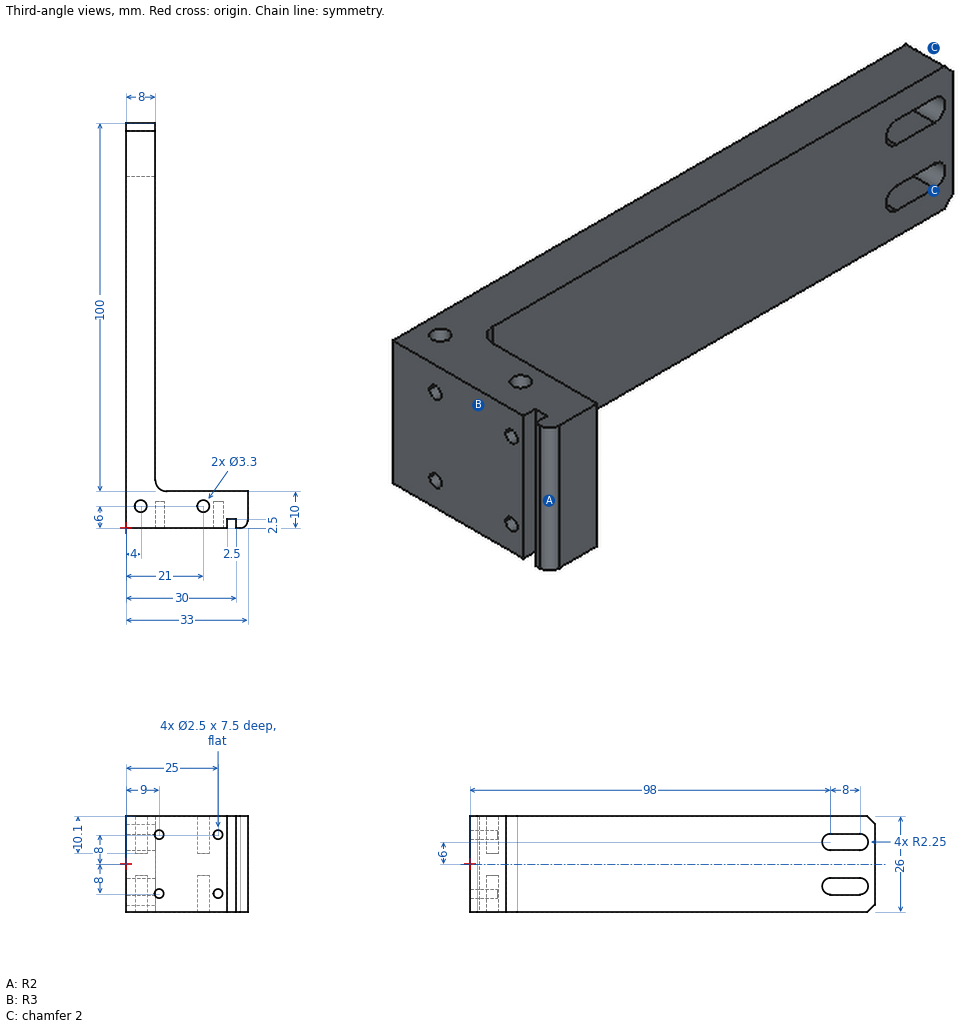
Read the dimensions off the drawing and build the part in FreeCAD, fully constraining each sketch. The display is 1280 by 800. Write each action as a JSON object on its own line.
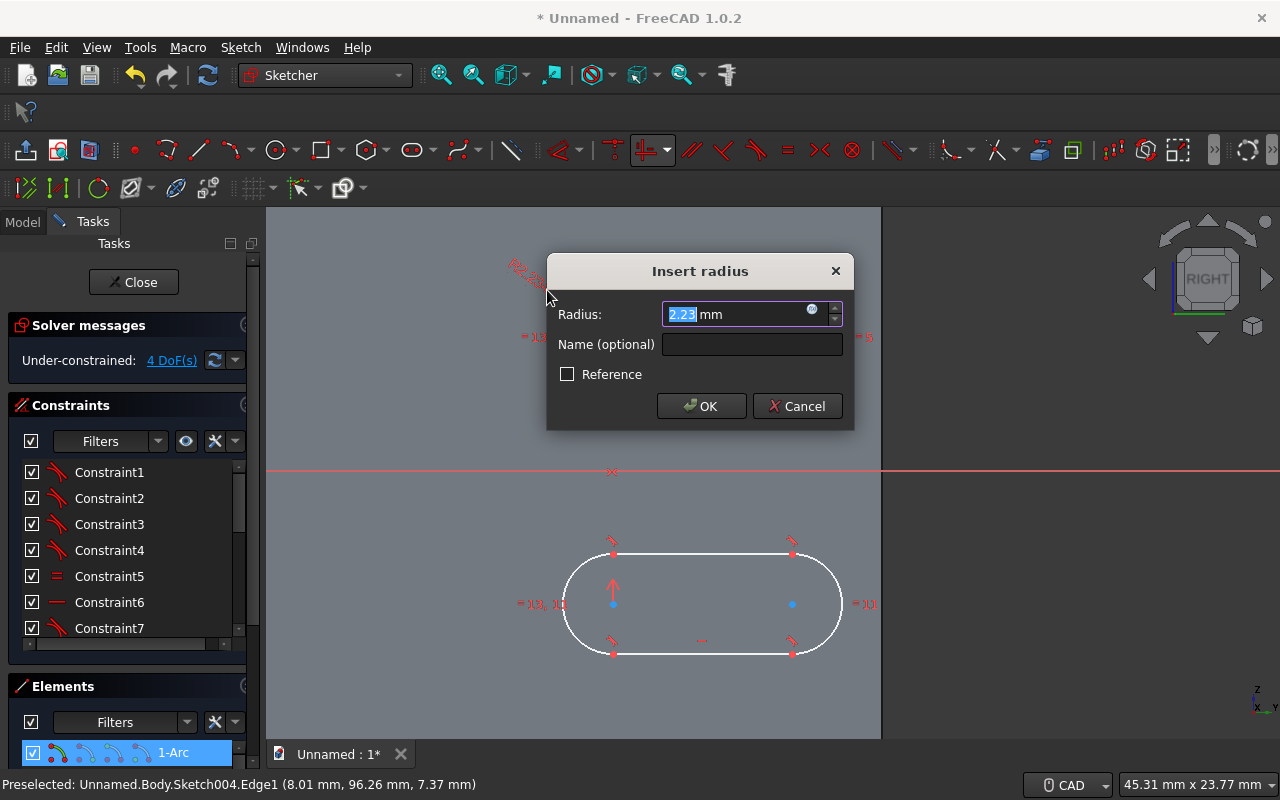
{"action": "type", "text": "2.25"}
{"action": "key", "text": "Return"}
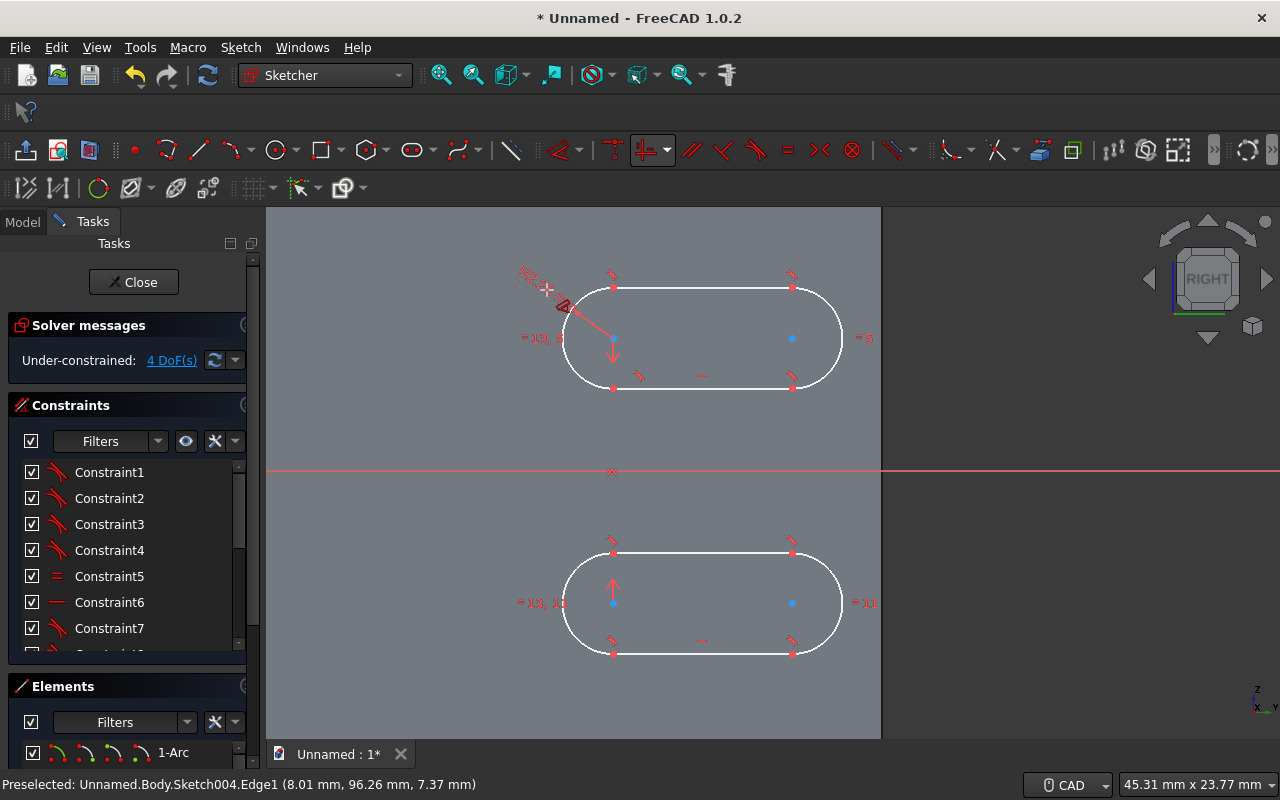
{"action": "left_click", "coordinate": [667, 288]}
{"action": "left_click", "coordinate": [702, 254]}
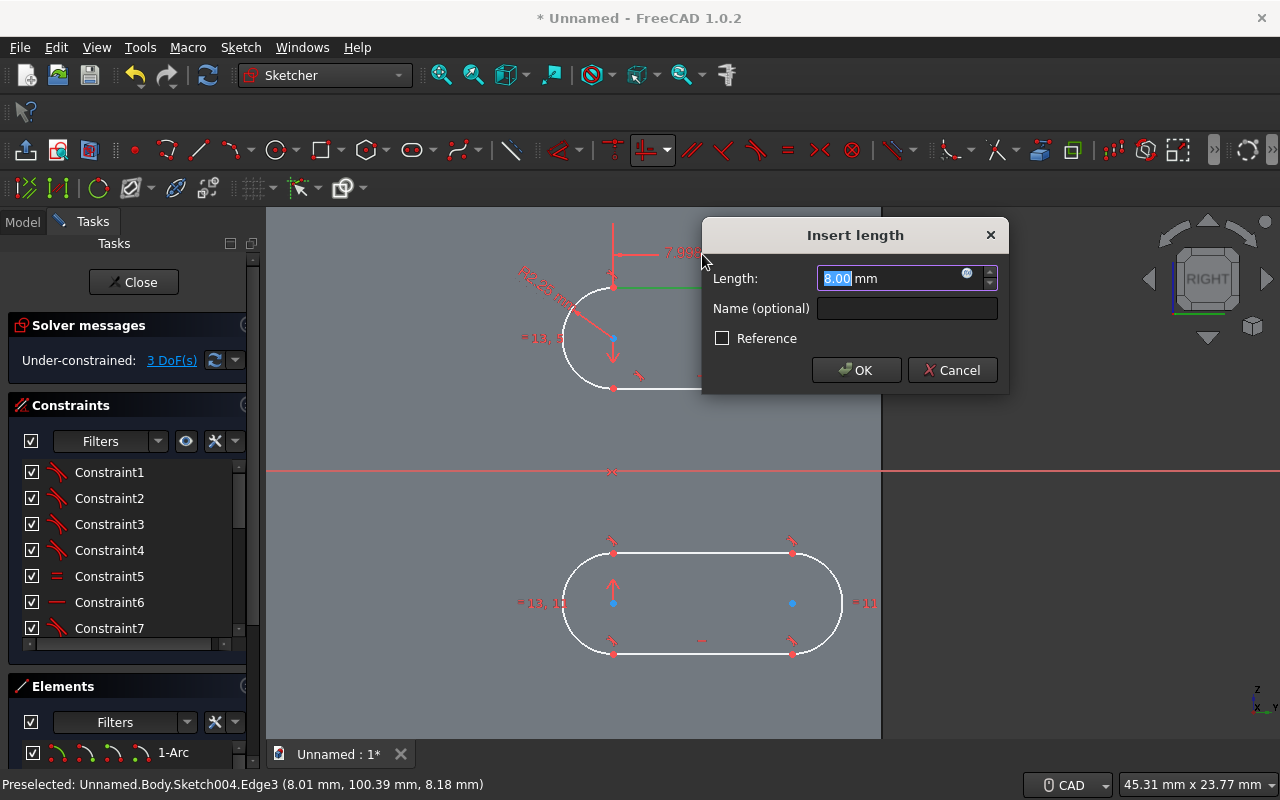
{"action": "type", "text": "8"}
{"action": "key", "text": "Return"}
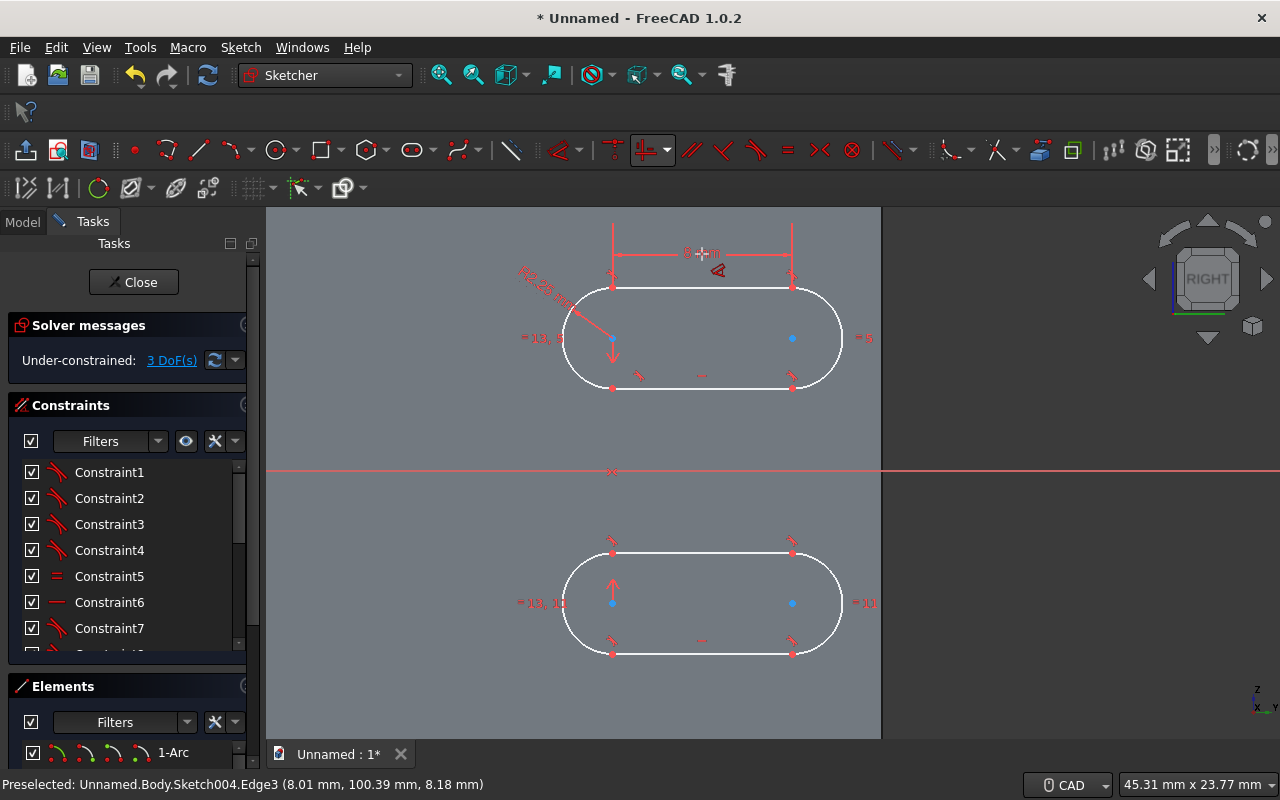
{"action": "left_click", "coordinate": [667, 553]}
{"action": "left_click", "coordinate": [702, 587]}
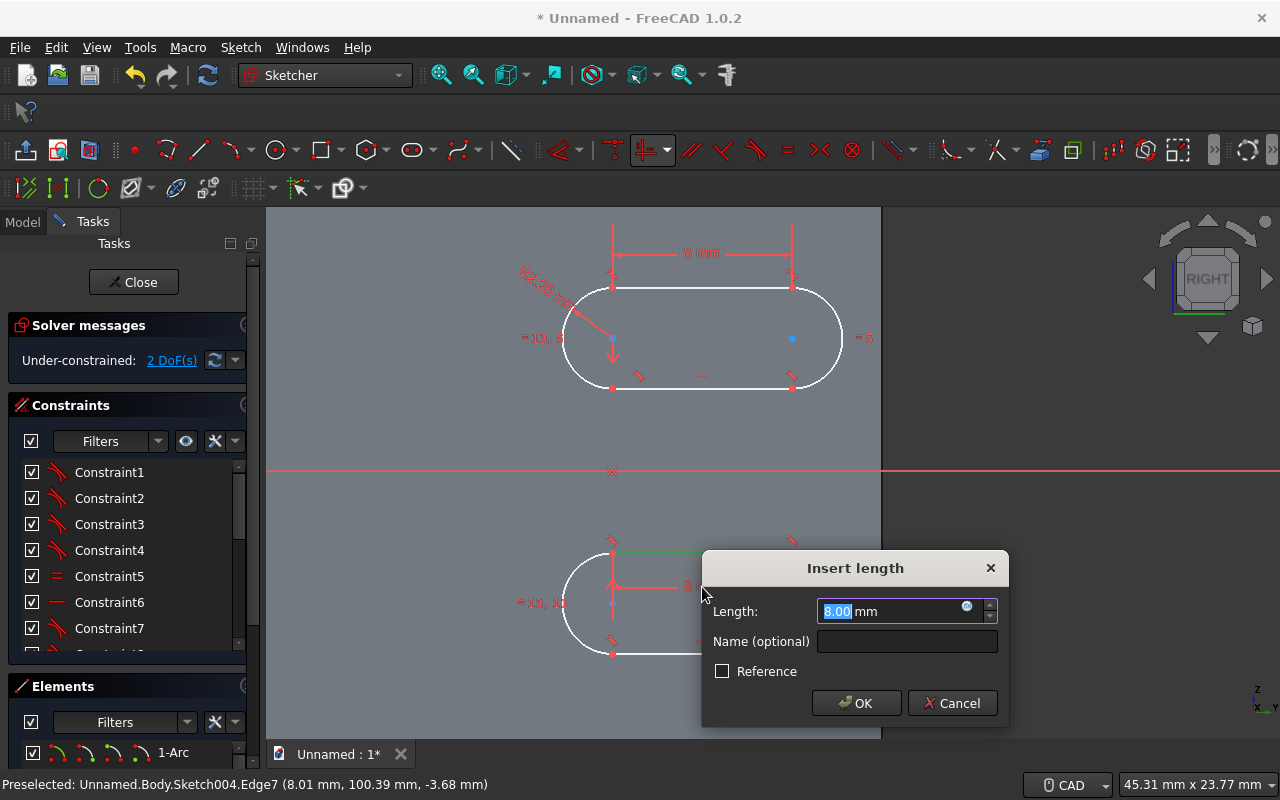
{"action": "type", "text": "8"}
{"action": "key", "text": "Return"}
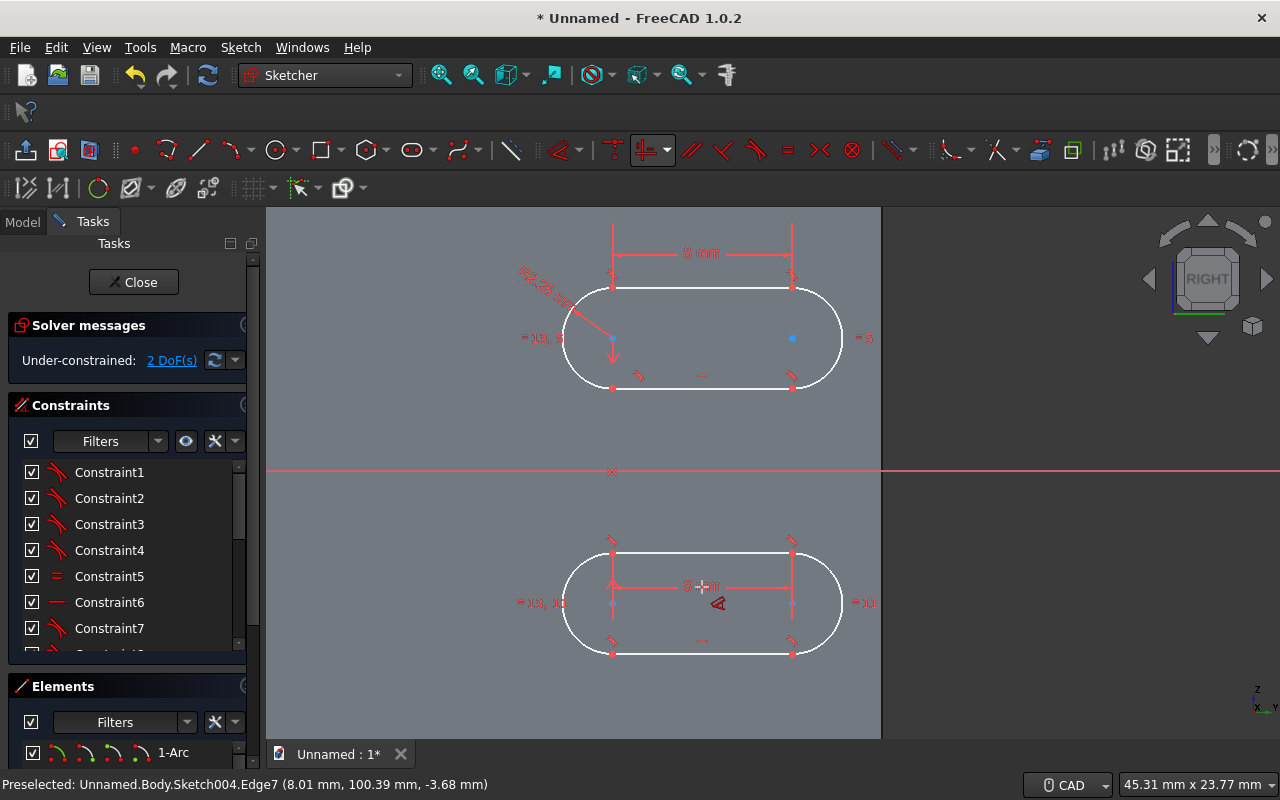
{"action": "left_click", "coordinate": [613, 338]}
{"action": "left_click", "coordinate": [647, 405]}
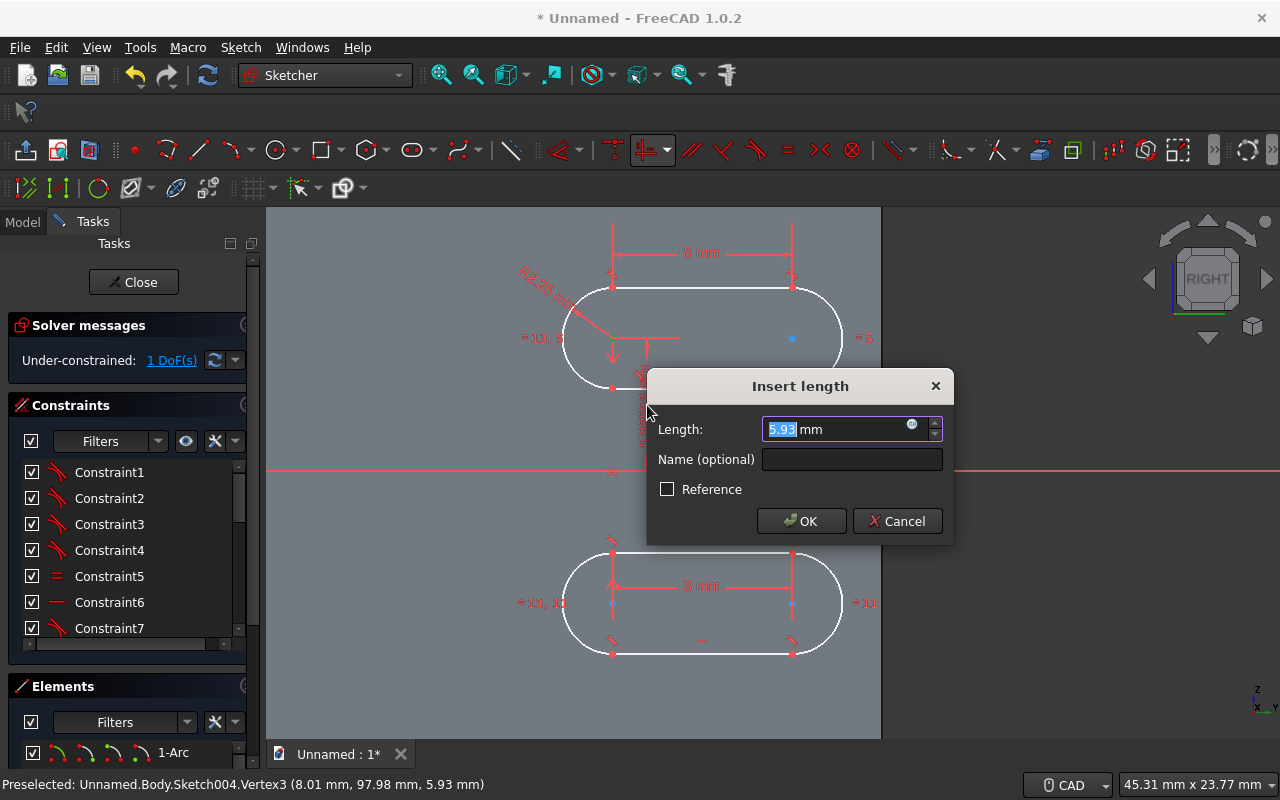
{"action": "type", "text": "6"}
{"action": "key", "text": "Return"}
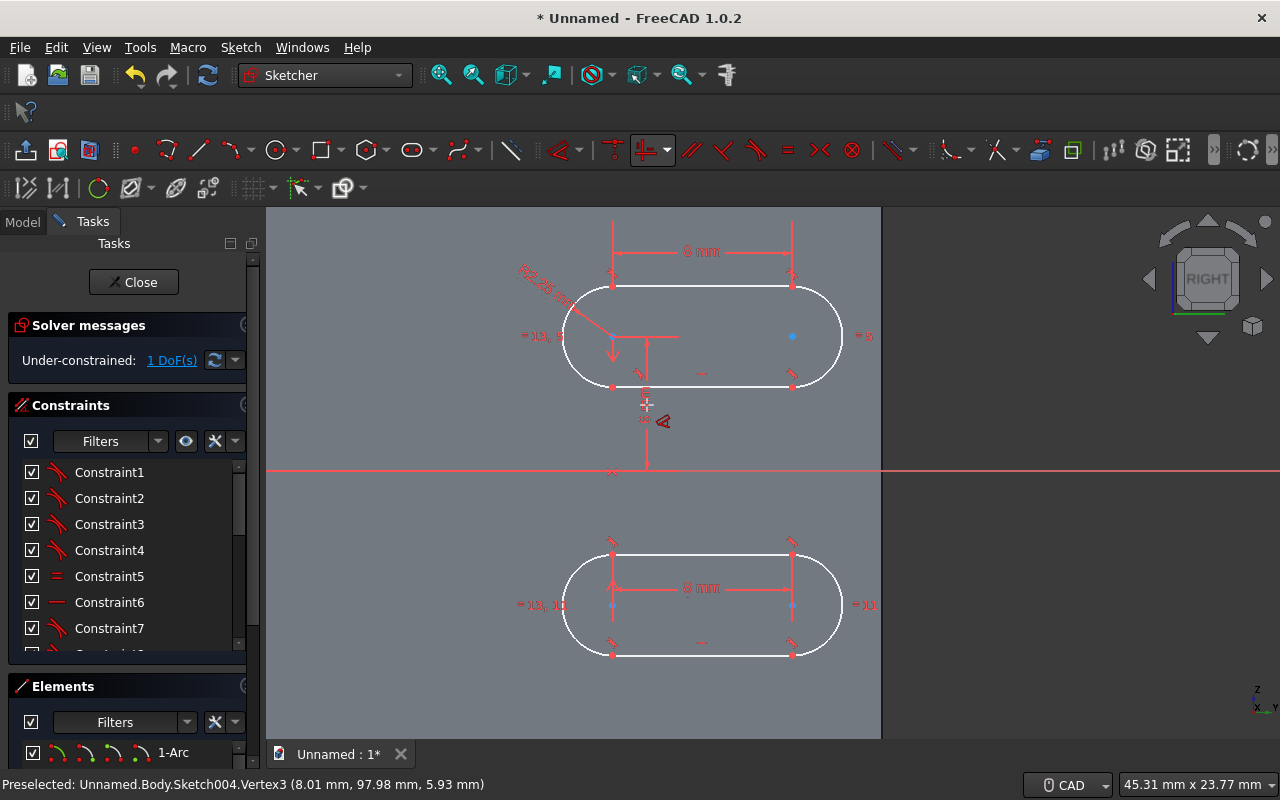
{"action": "left_click", "coordinate": [613, 286]}
{"action": "left_click", "coordinate": [453, 252]}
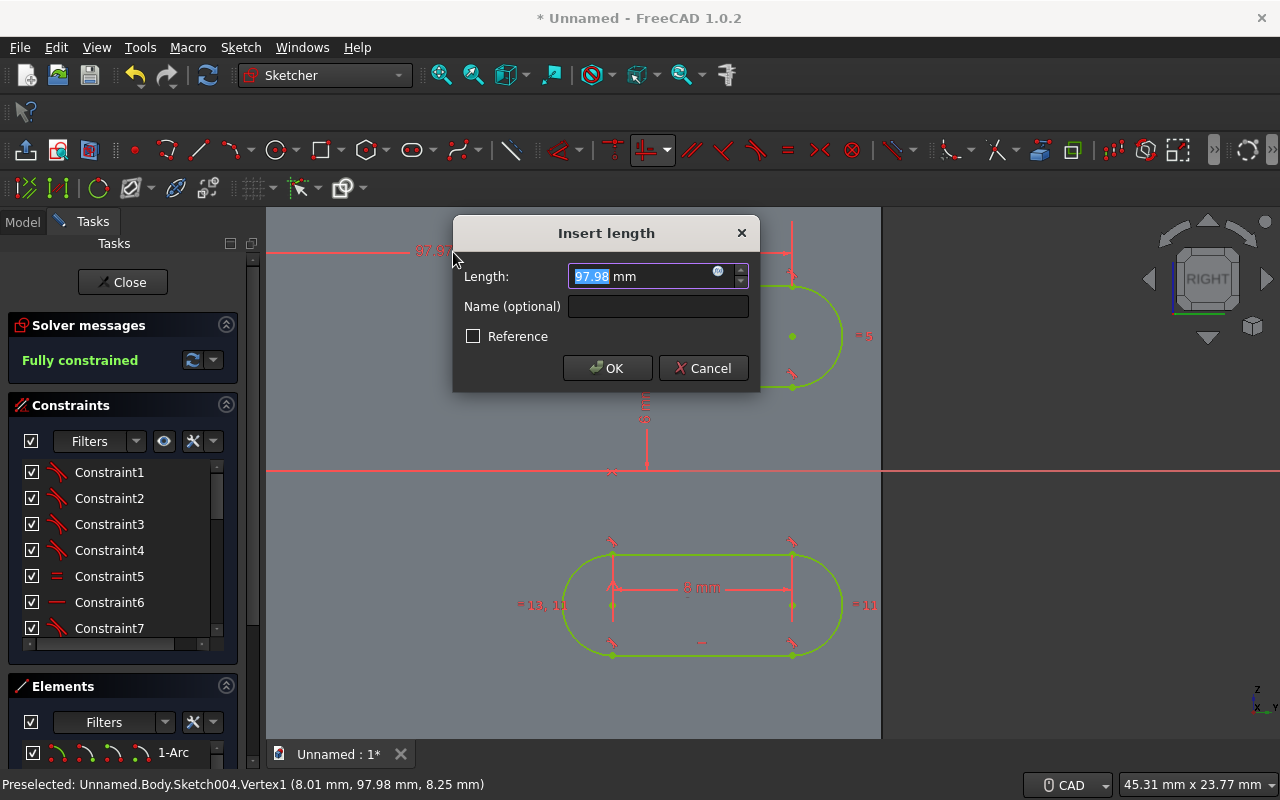
{"action": "type", "text": "98"}
{"action": "key", "text": "Return"}
{"action": "key", "text": "Escape"}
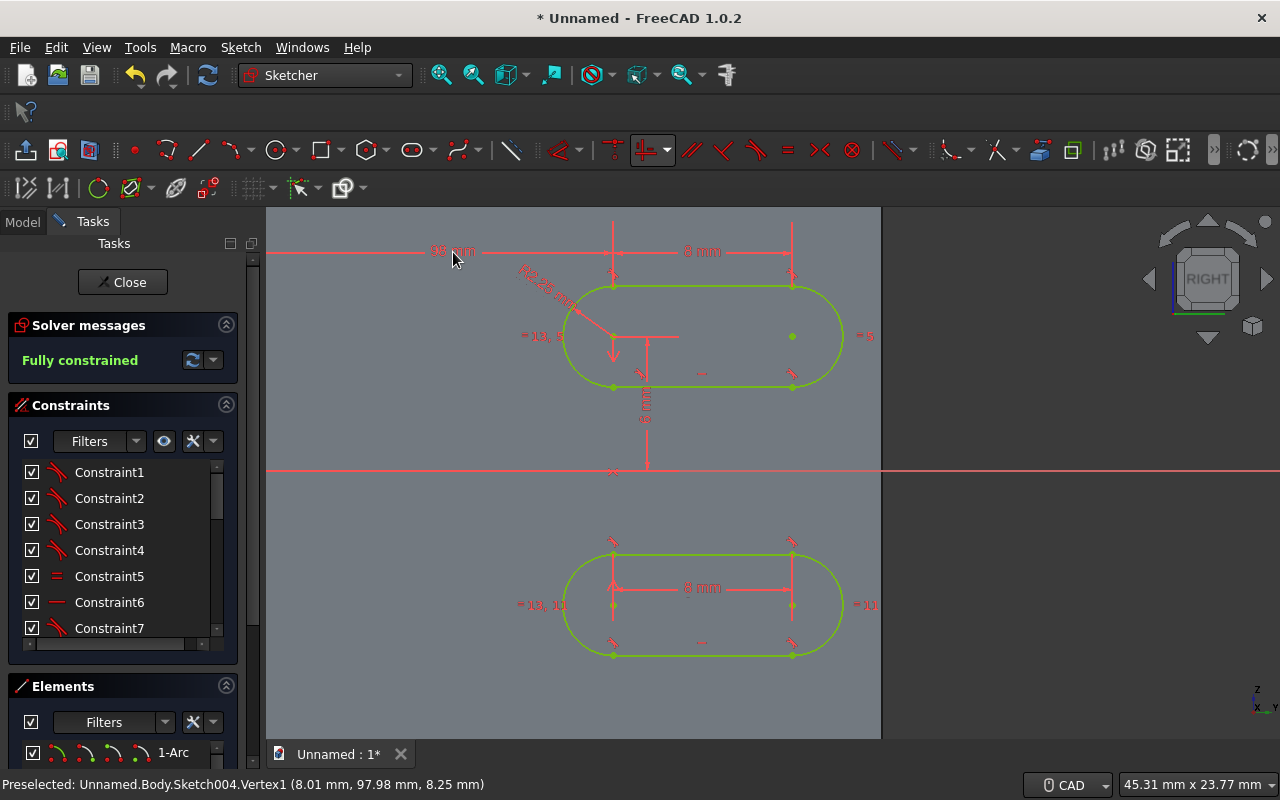
{"action": "left_click", "coordinate": [123, 282]}